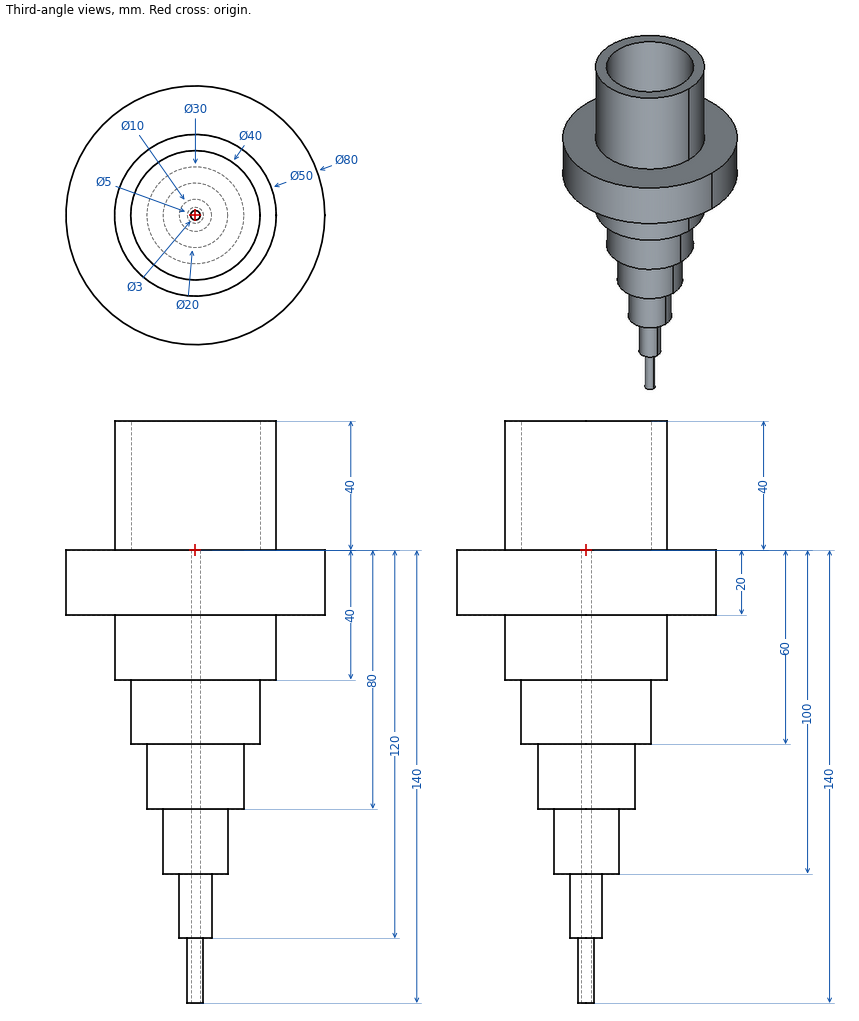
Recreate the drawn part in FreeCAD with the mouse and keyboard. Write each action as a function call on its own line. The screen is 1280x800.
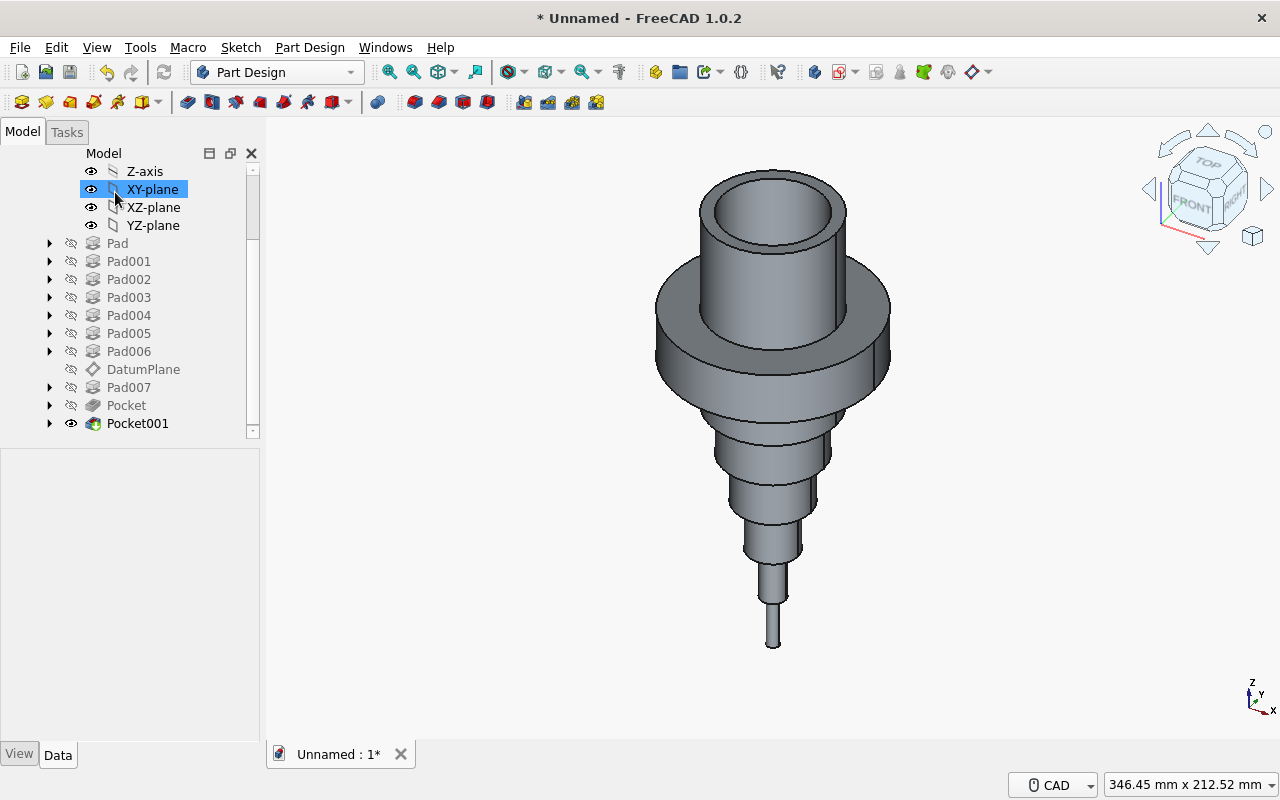
key(0)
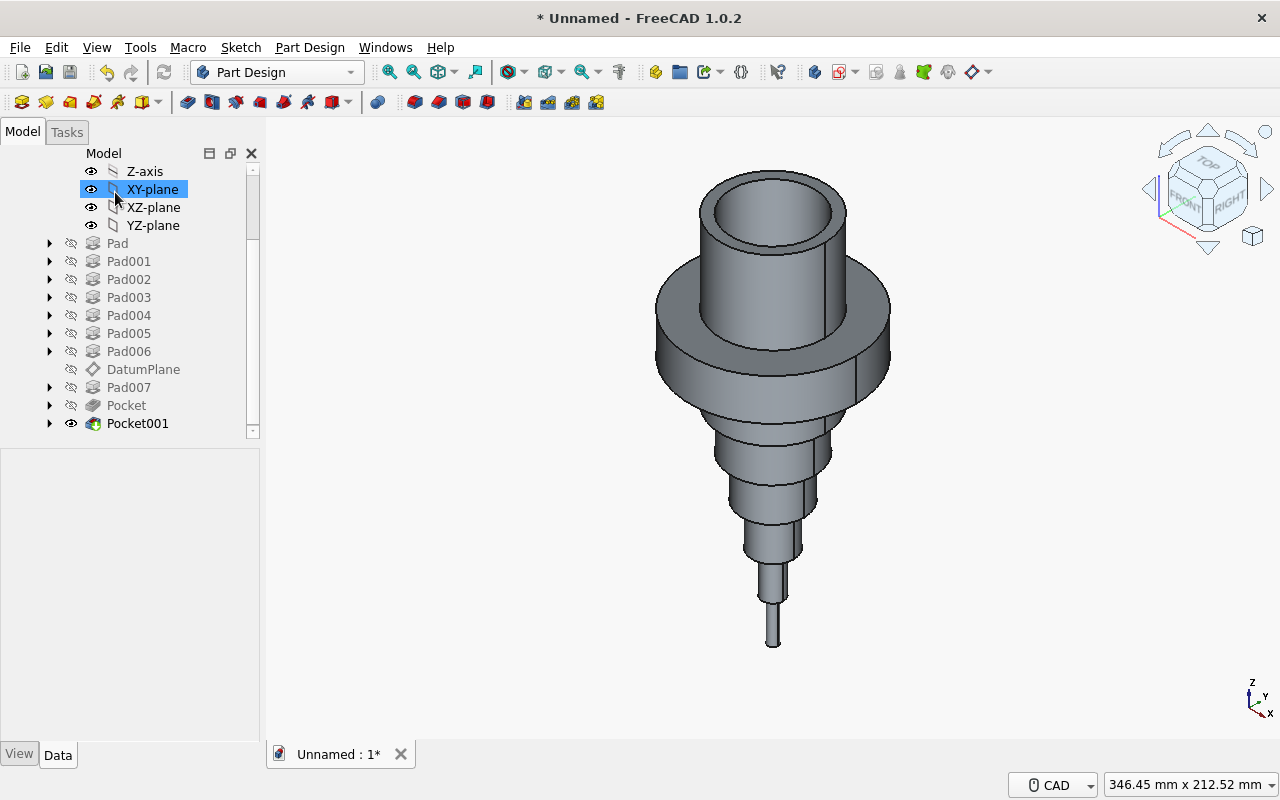
click(390, 72)